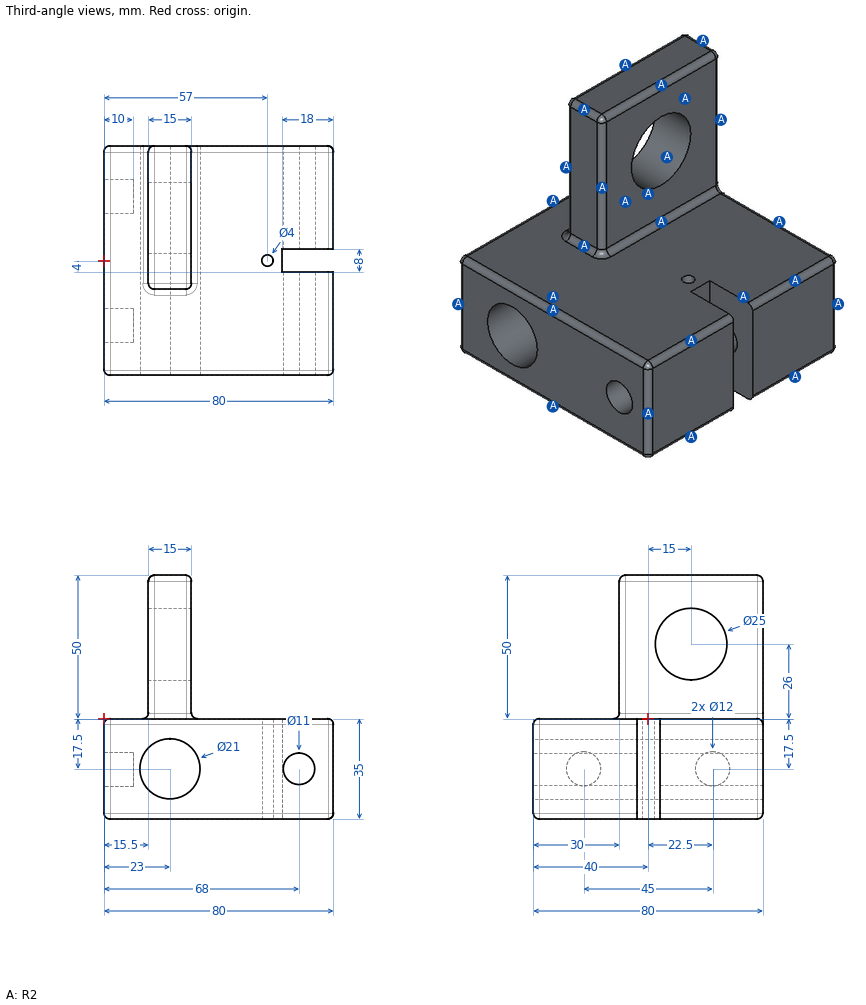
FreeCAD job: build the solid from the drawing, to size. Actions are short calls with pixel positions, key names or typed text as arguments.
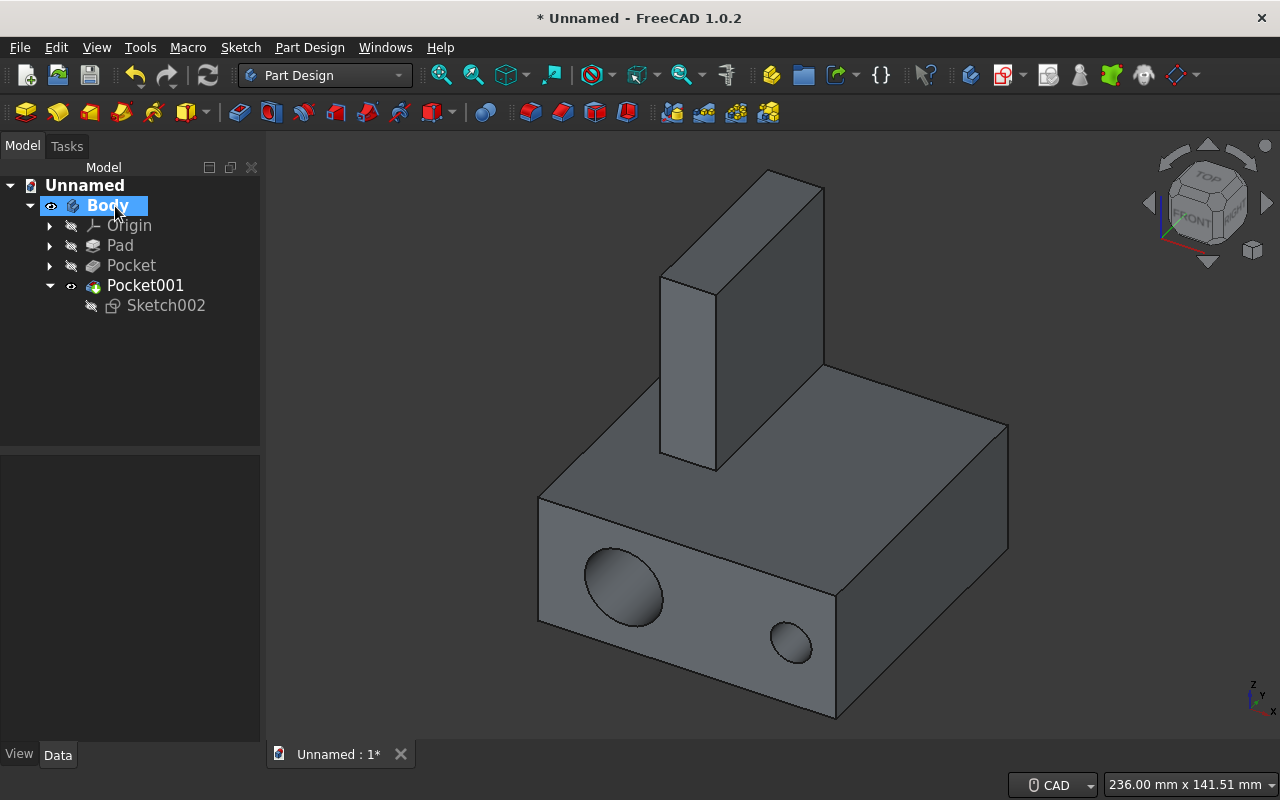
click(770, 329)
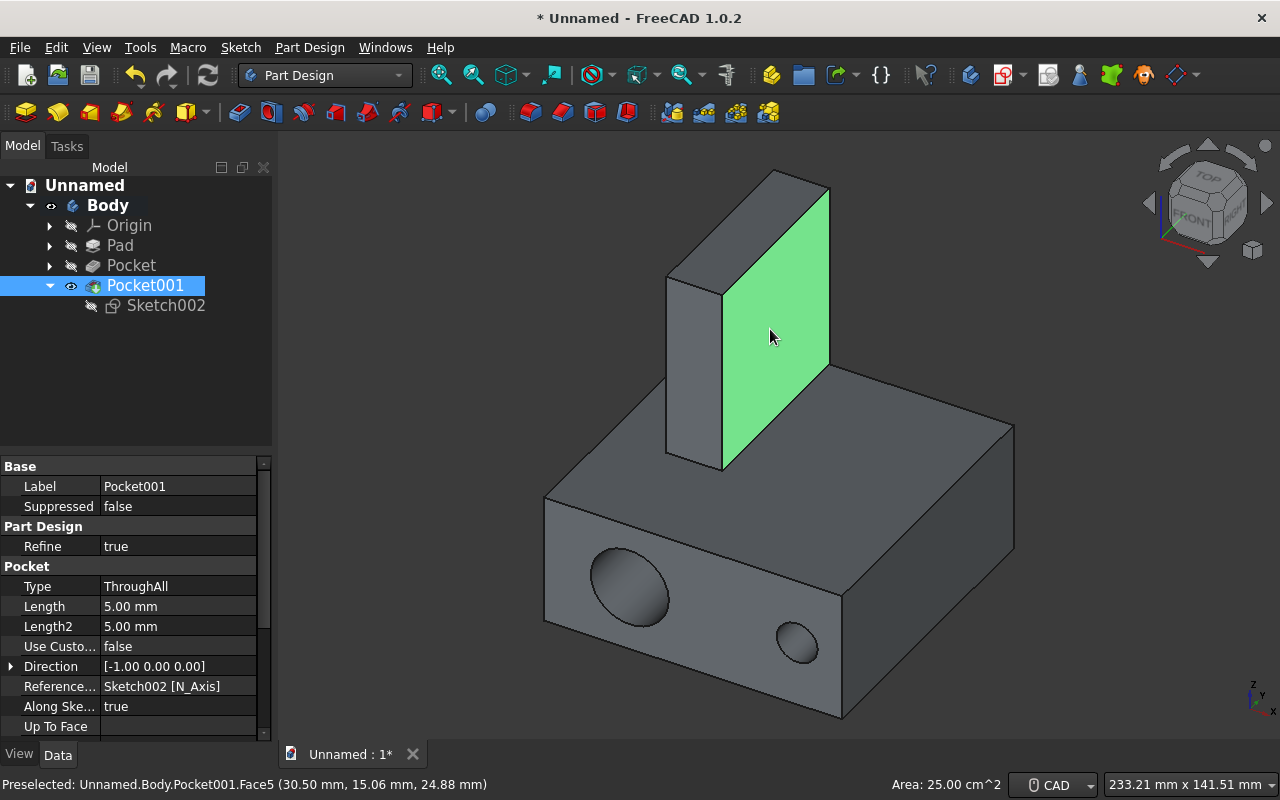
click(1004, 76)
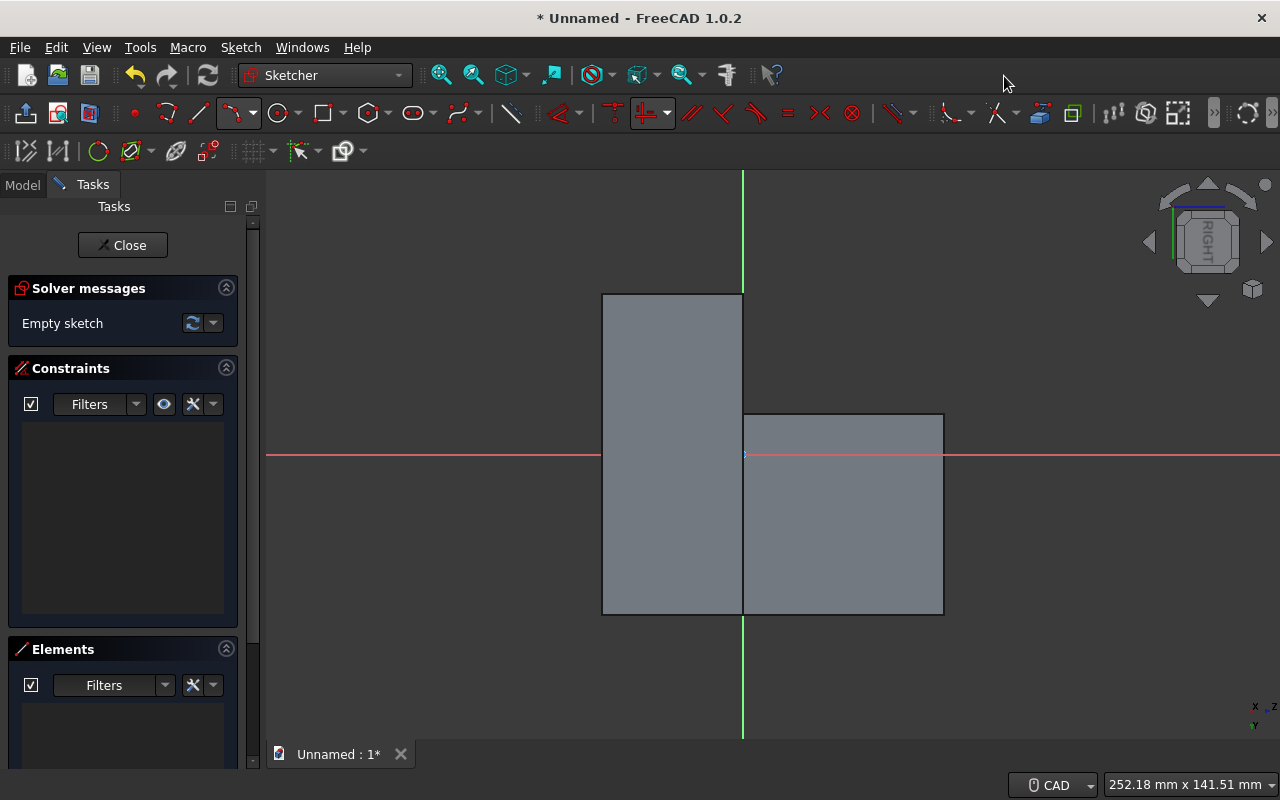
click(90, 114)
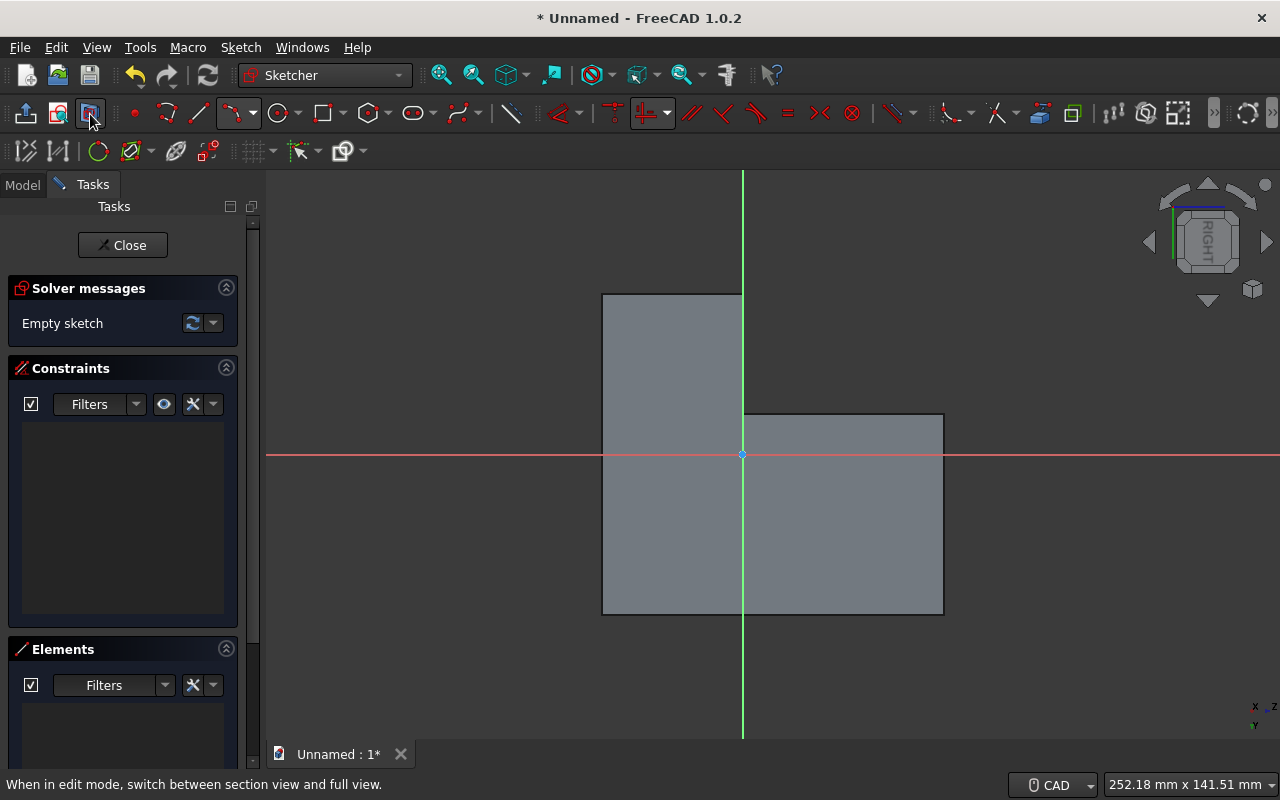
scroll(870, 534, up, 6)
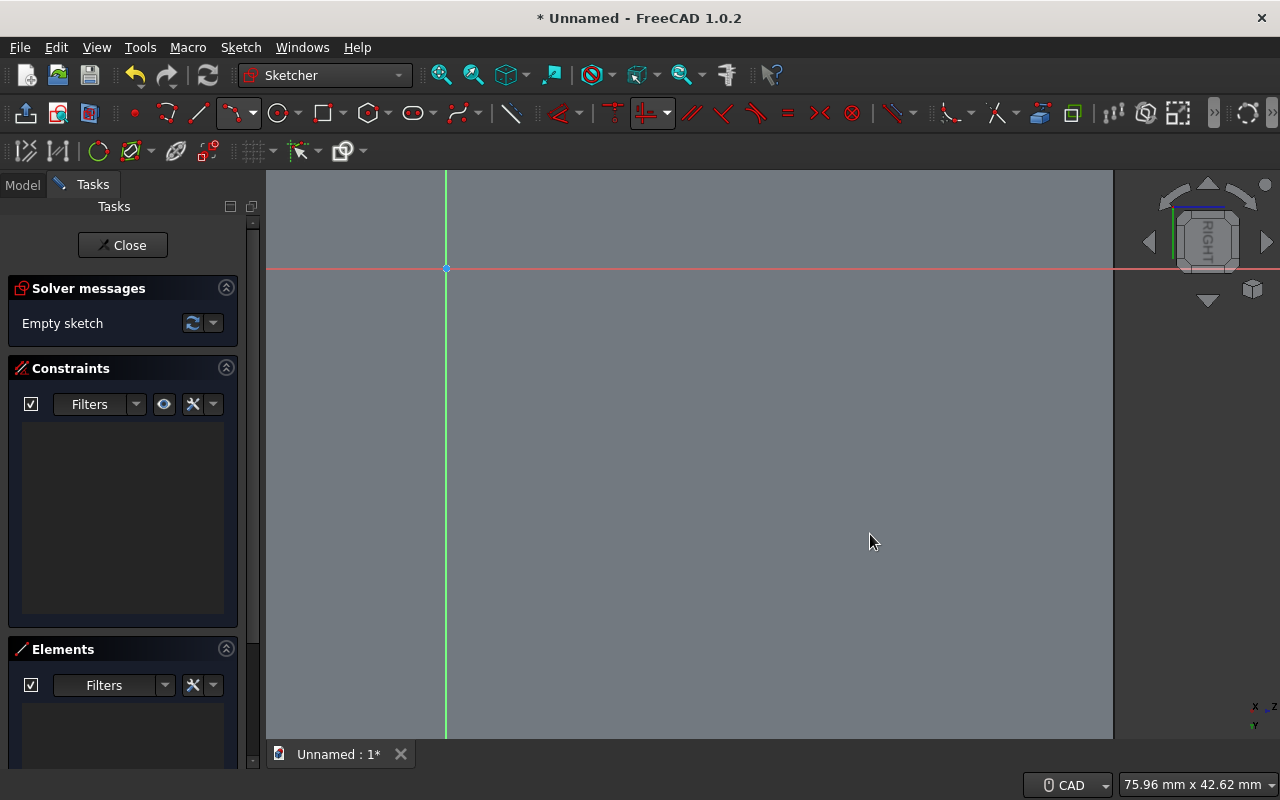
click(278, 114)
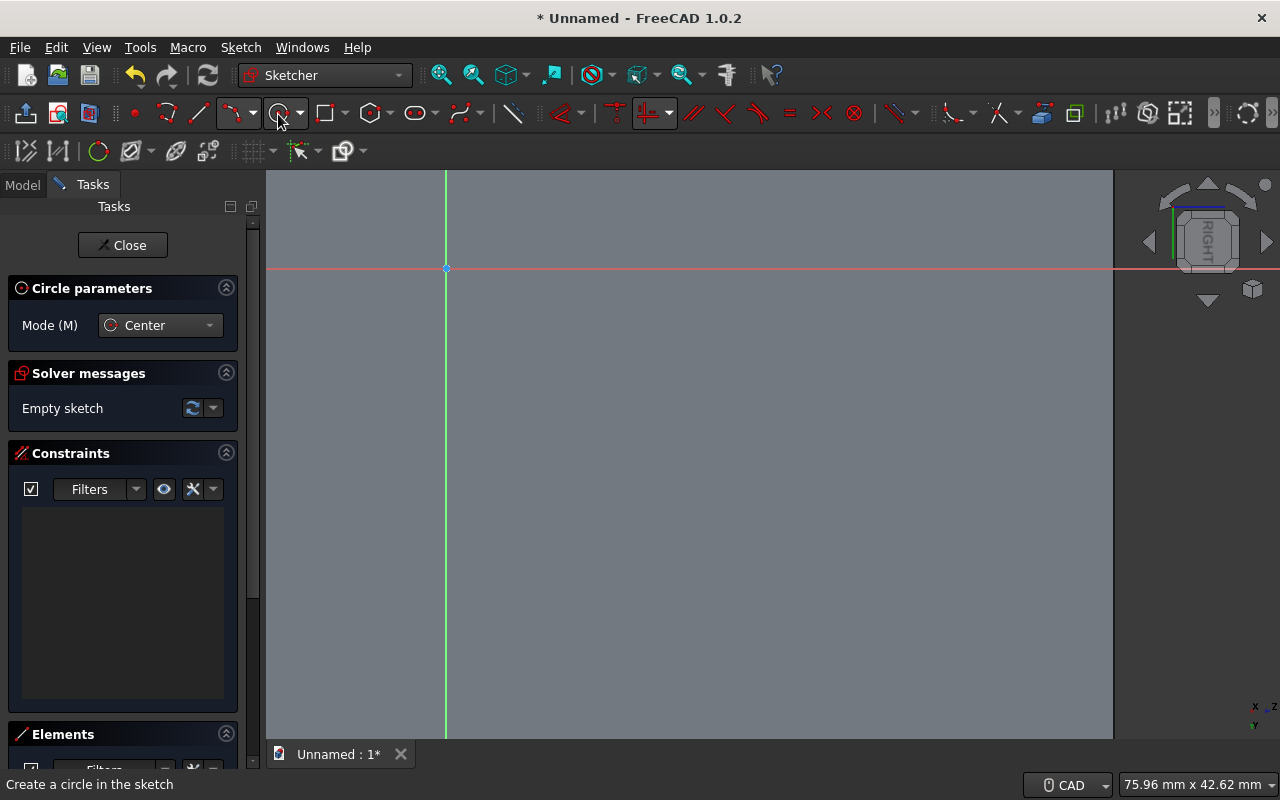
click(794, 469)
click(912, 351)
key(Escape)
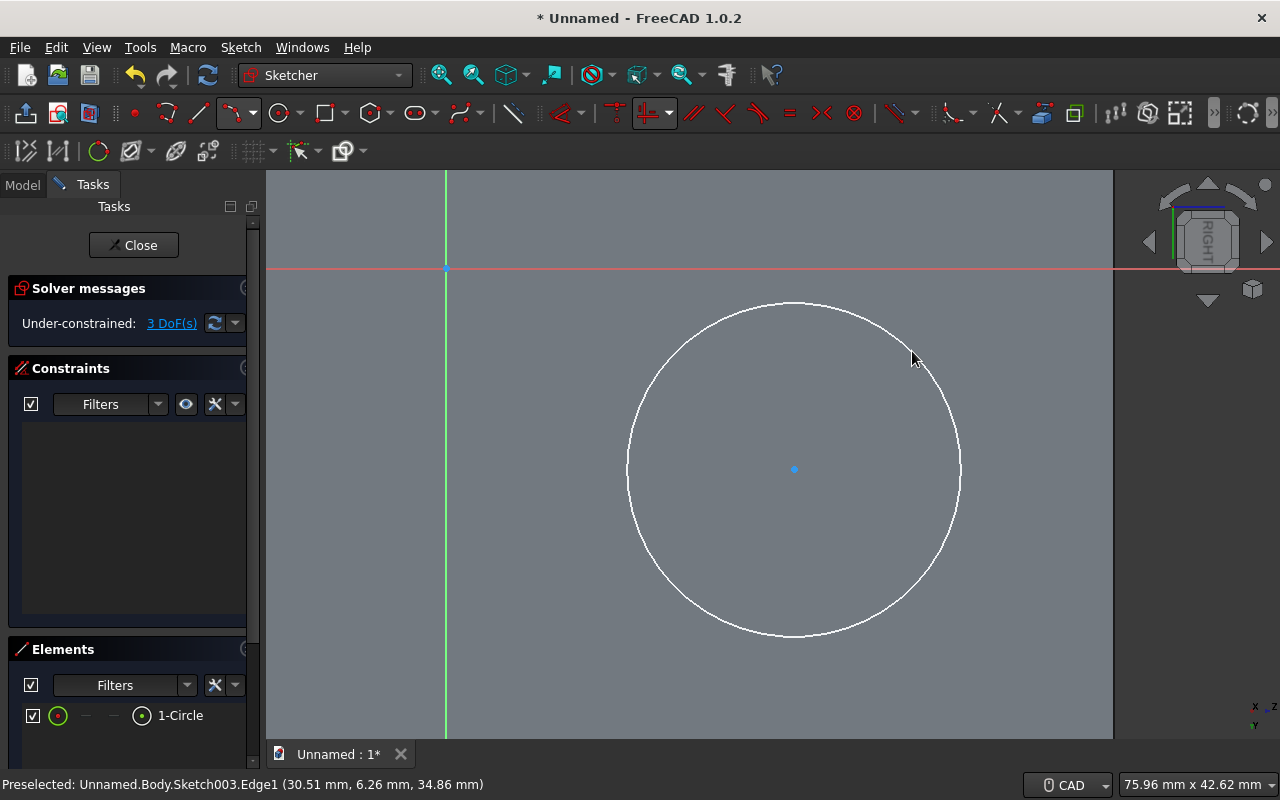
click(560, 114)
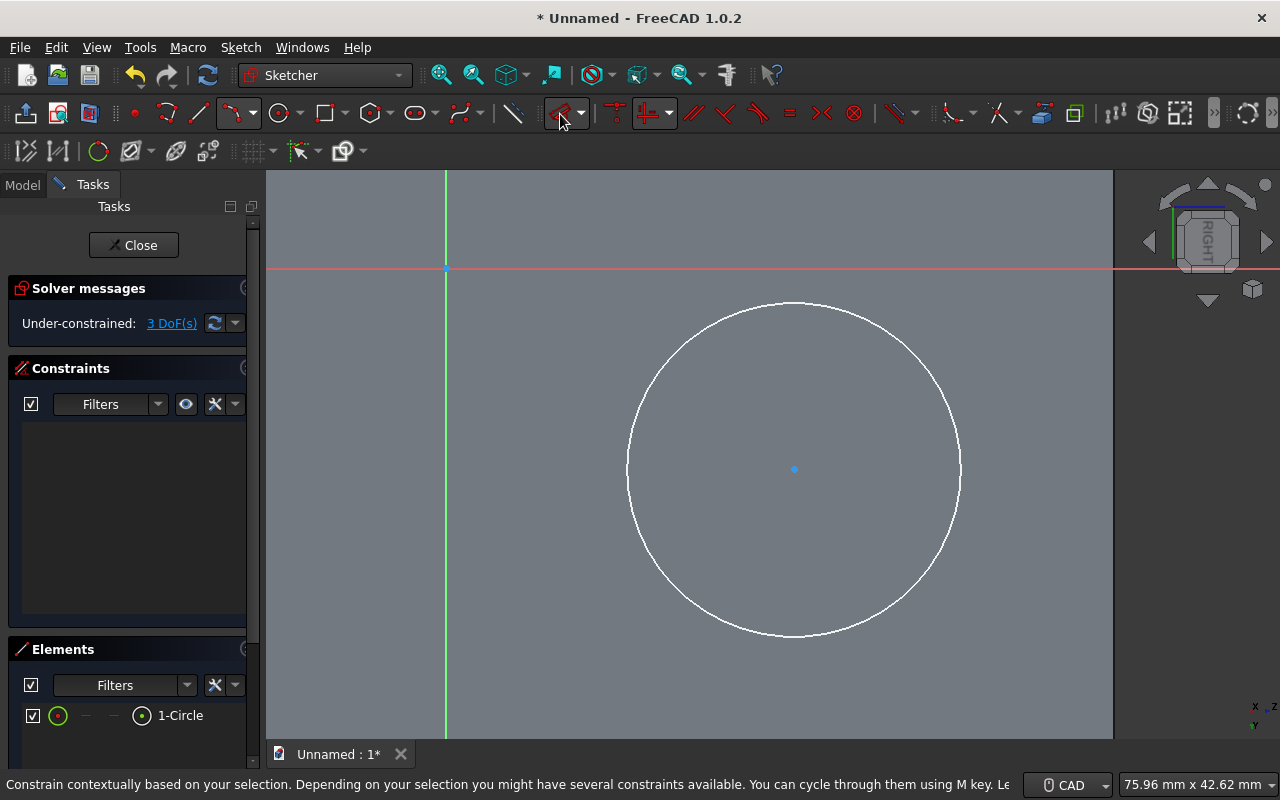
click(912, 352)
click(935, 329)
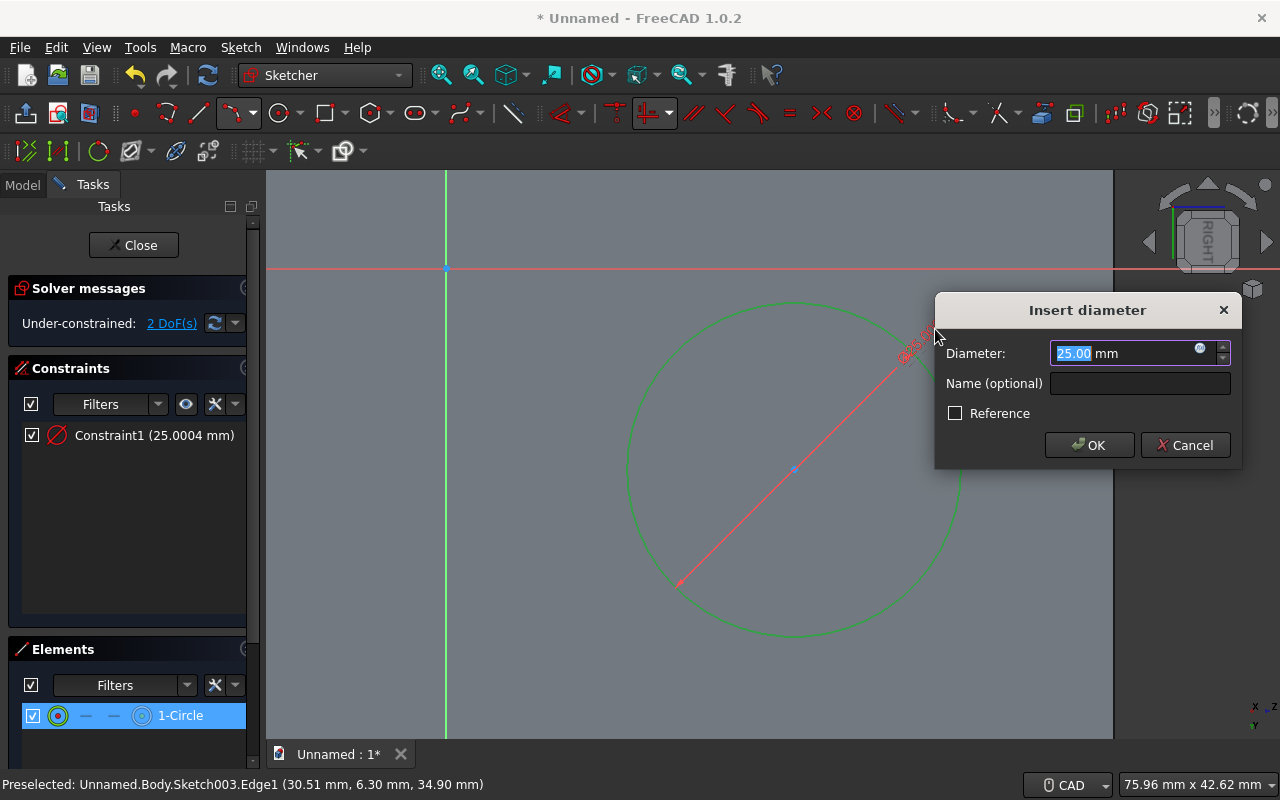
text(25)
key(Return)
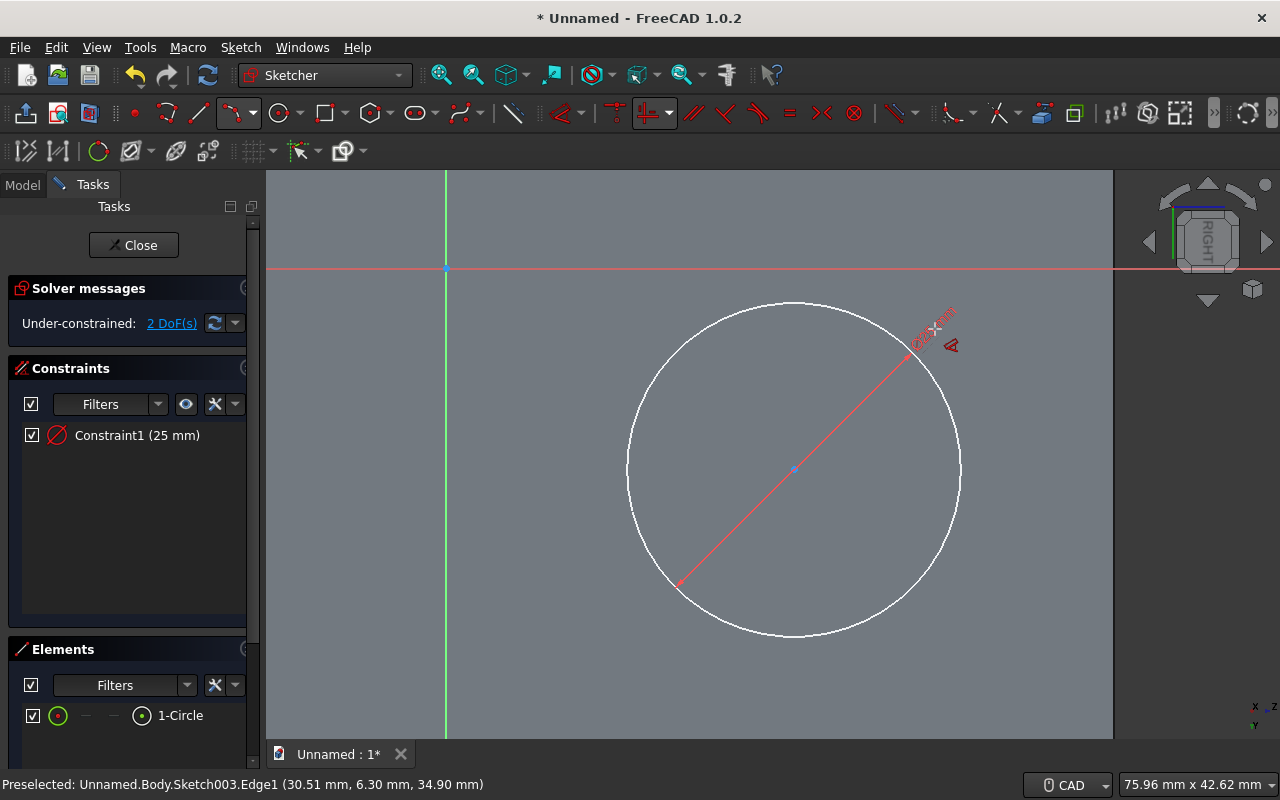
click(794, 470)
click(620, 235)